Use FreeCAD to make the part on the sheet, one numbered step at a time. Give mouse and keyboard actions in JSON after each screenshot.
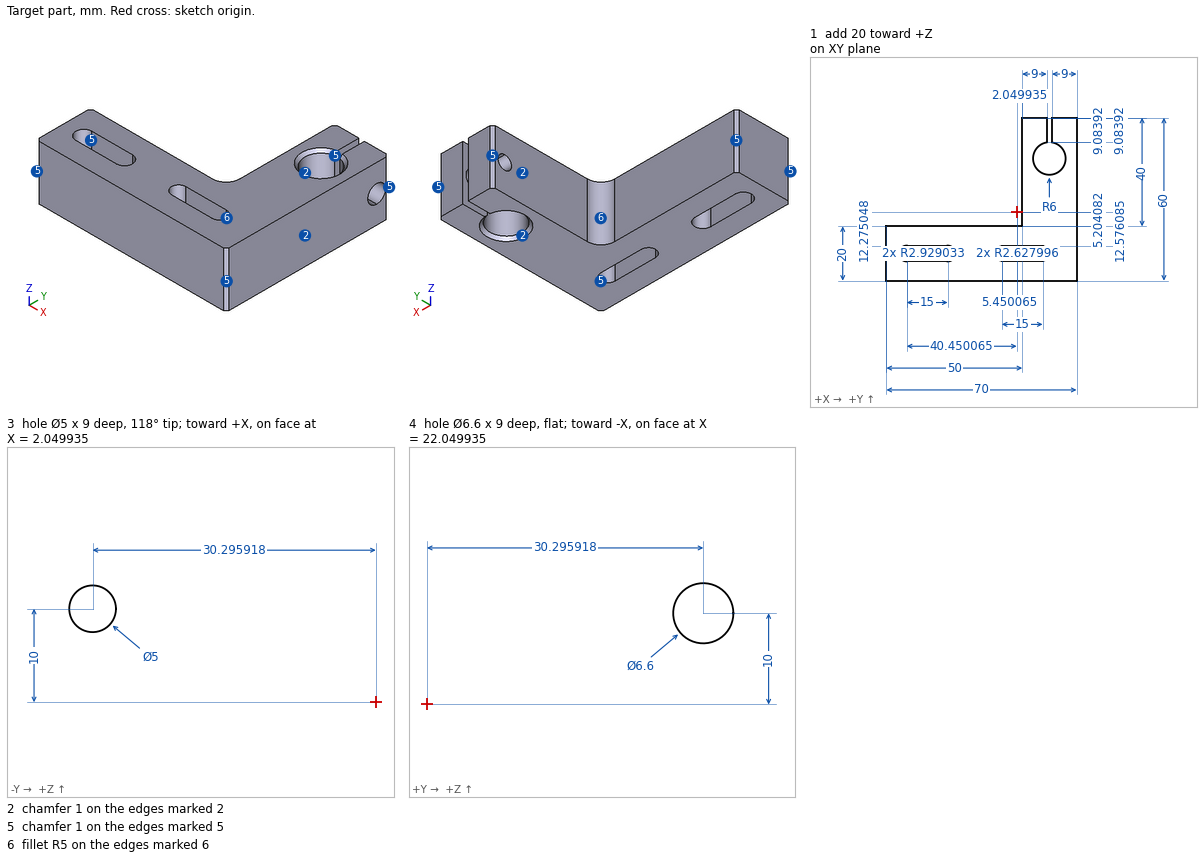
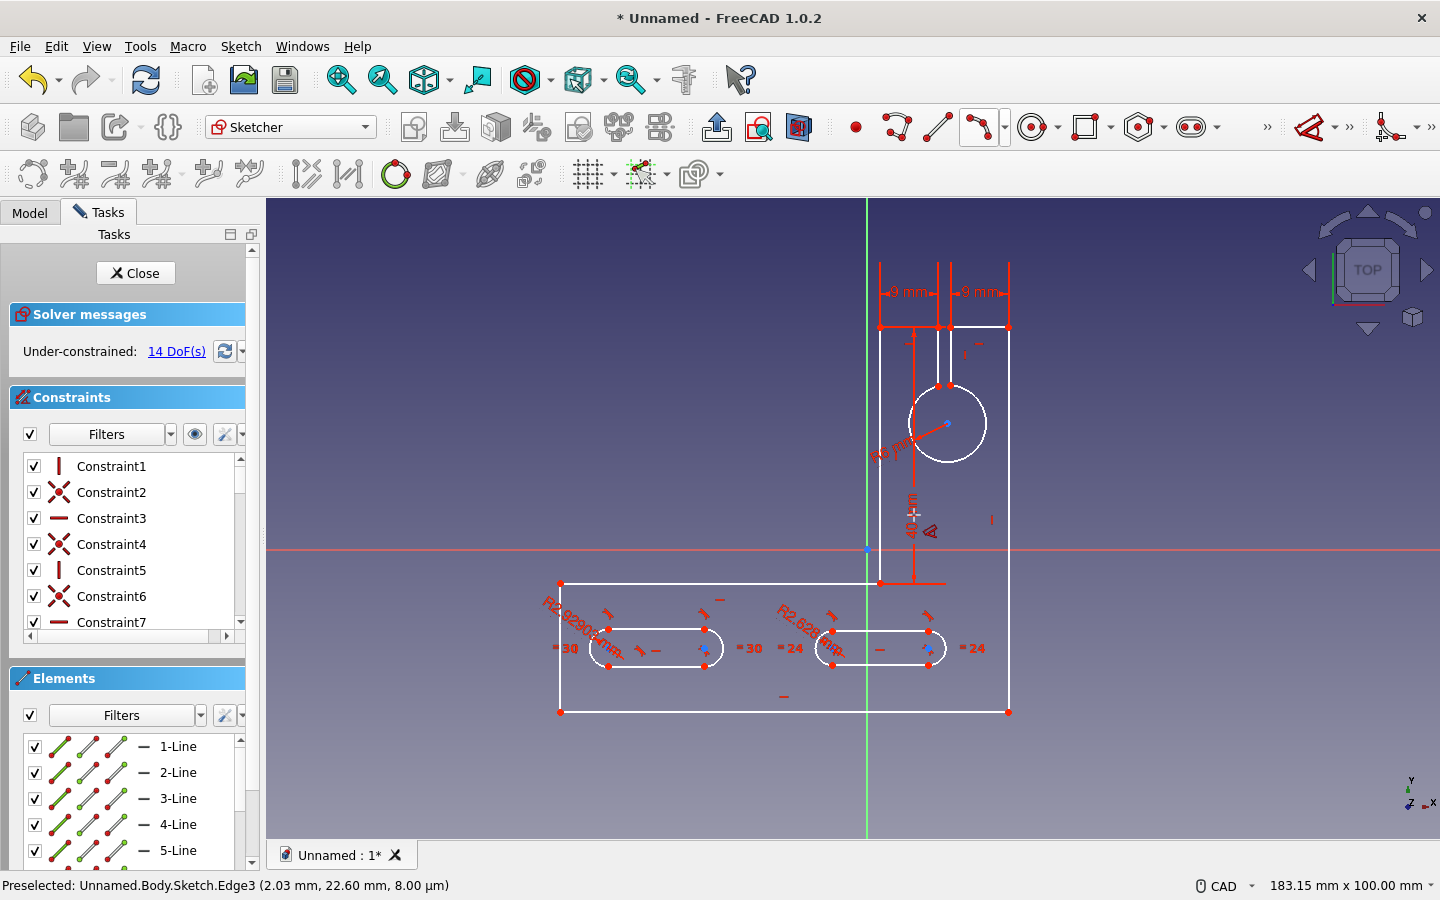
{"action": "left_click", "coordinate": [784, 584]}
{"action": "left_click", "coordinate": [720, 618]}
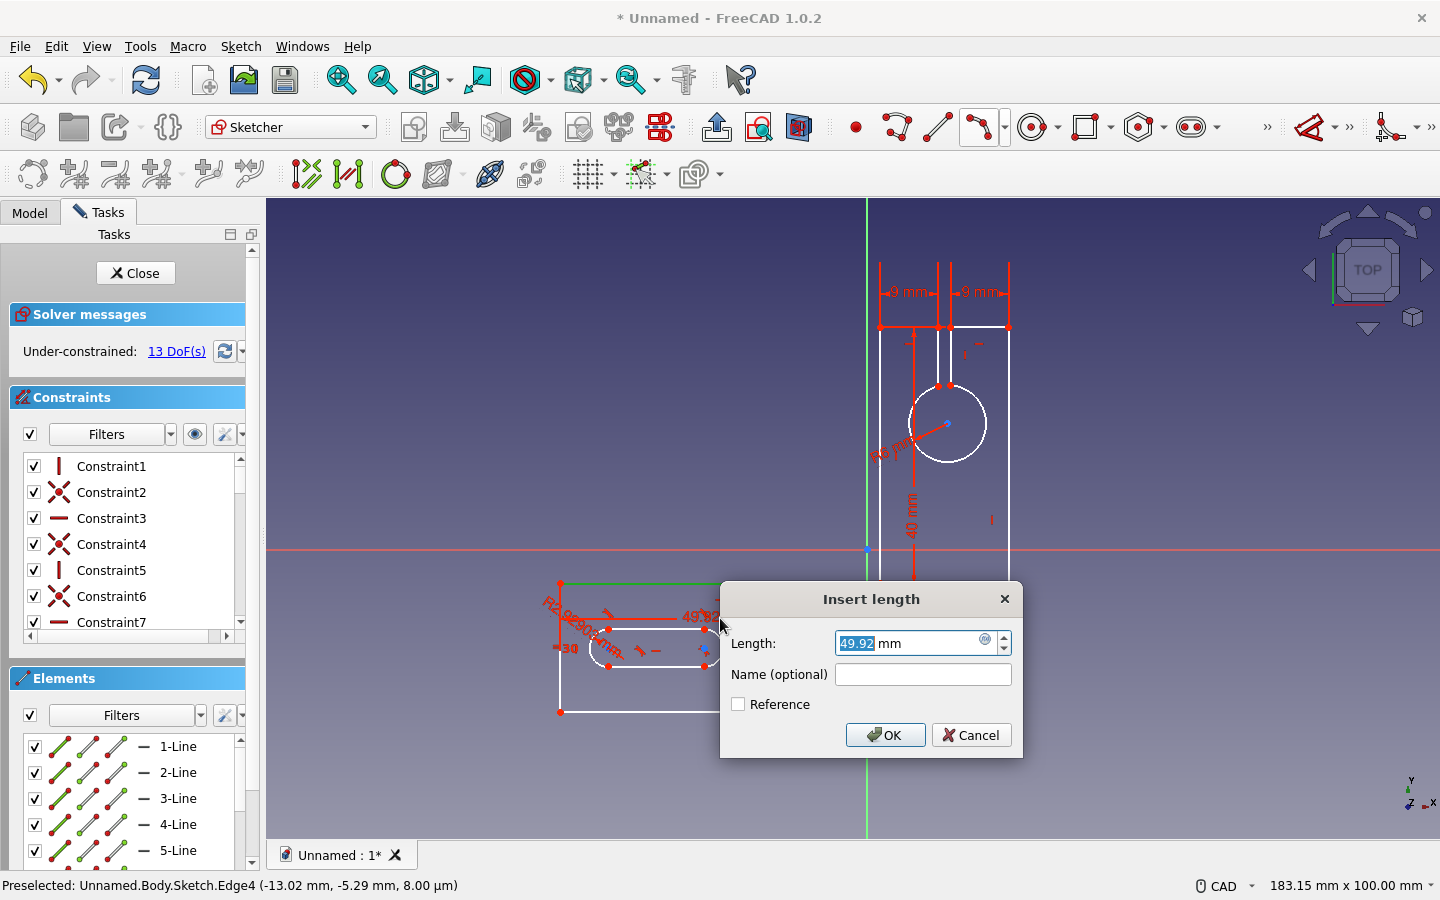
{"action": "type", "text": "50"}
{"action": "key", "text": "Return"}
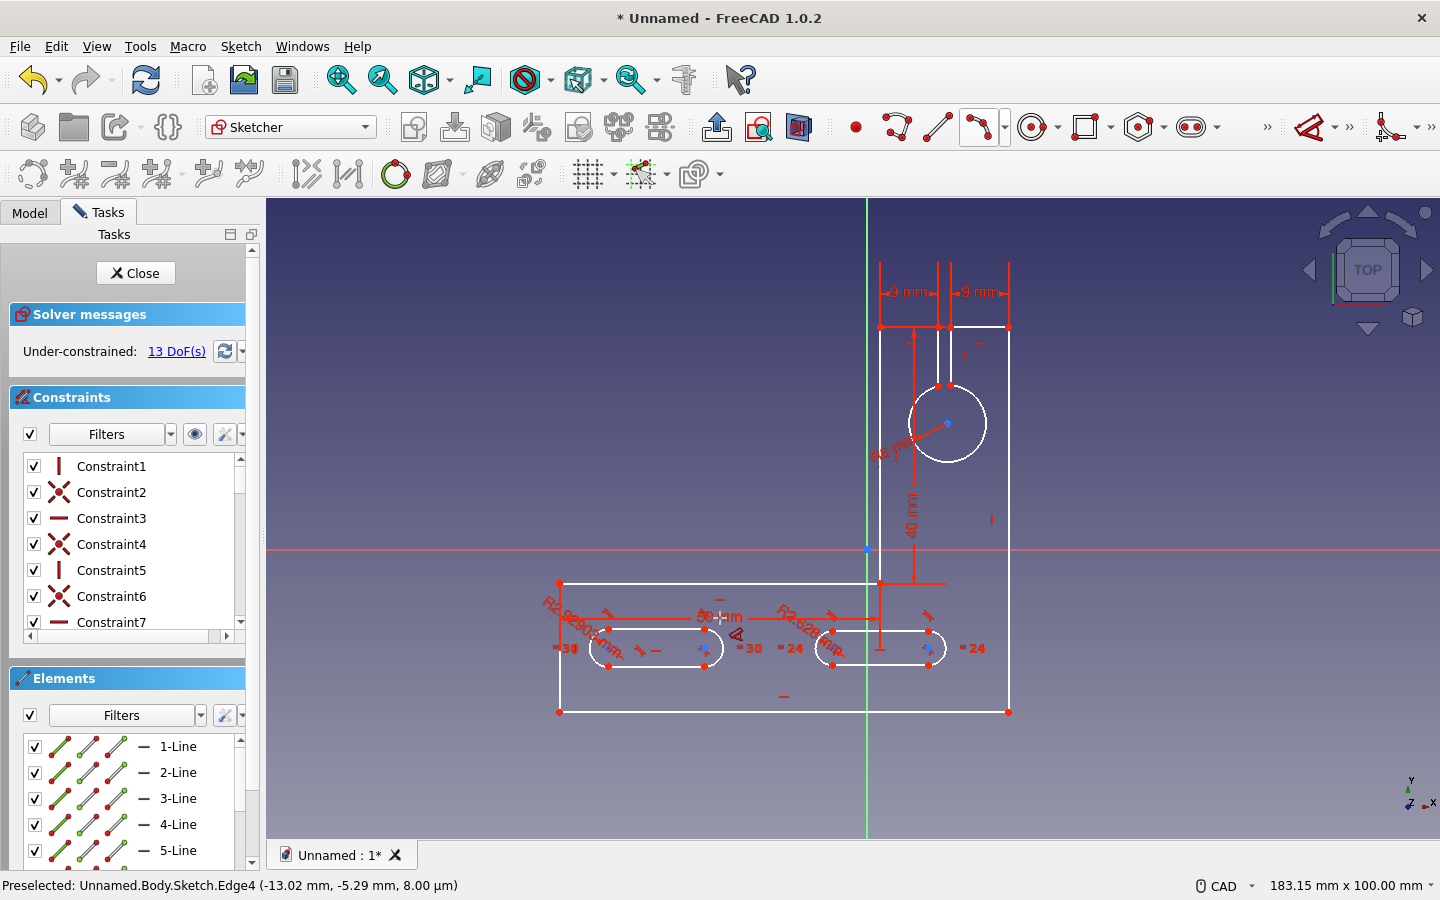
{"action": "left_click", "coordinate": [560, 622]}
{"action": "left_click", "coordinate": [526, 678]}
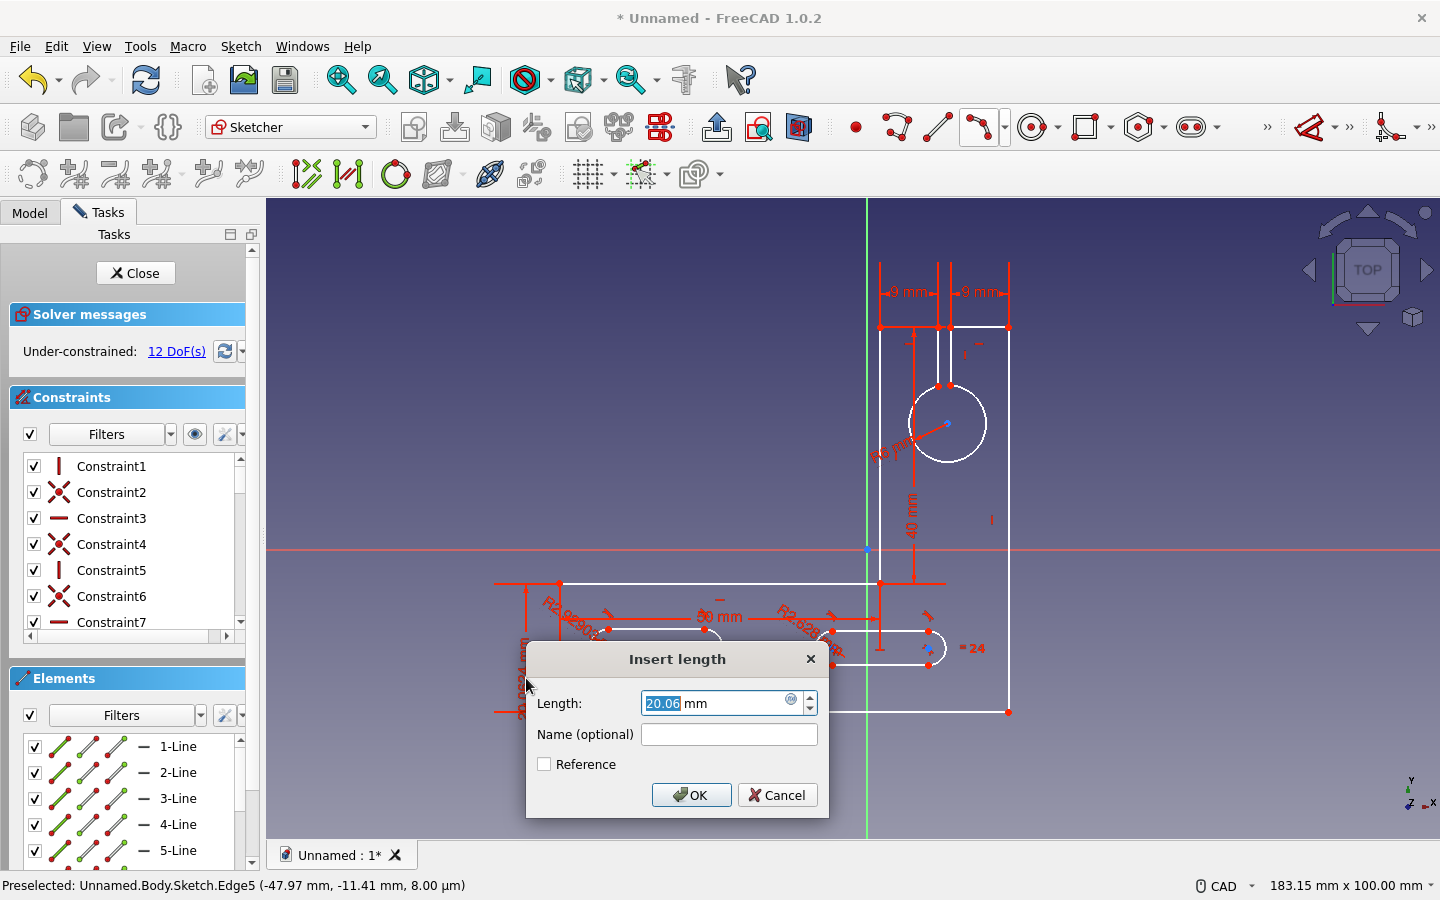
{"action": "type", "text": "20"}
{"action": "key", "text": "Return"}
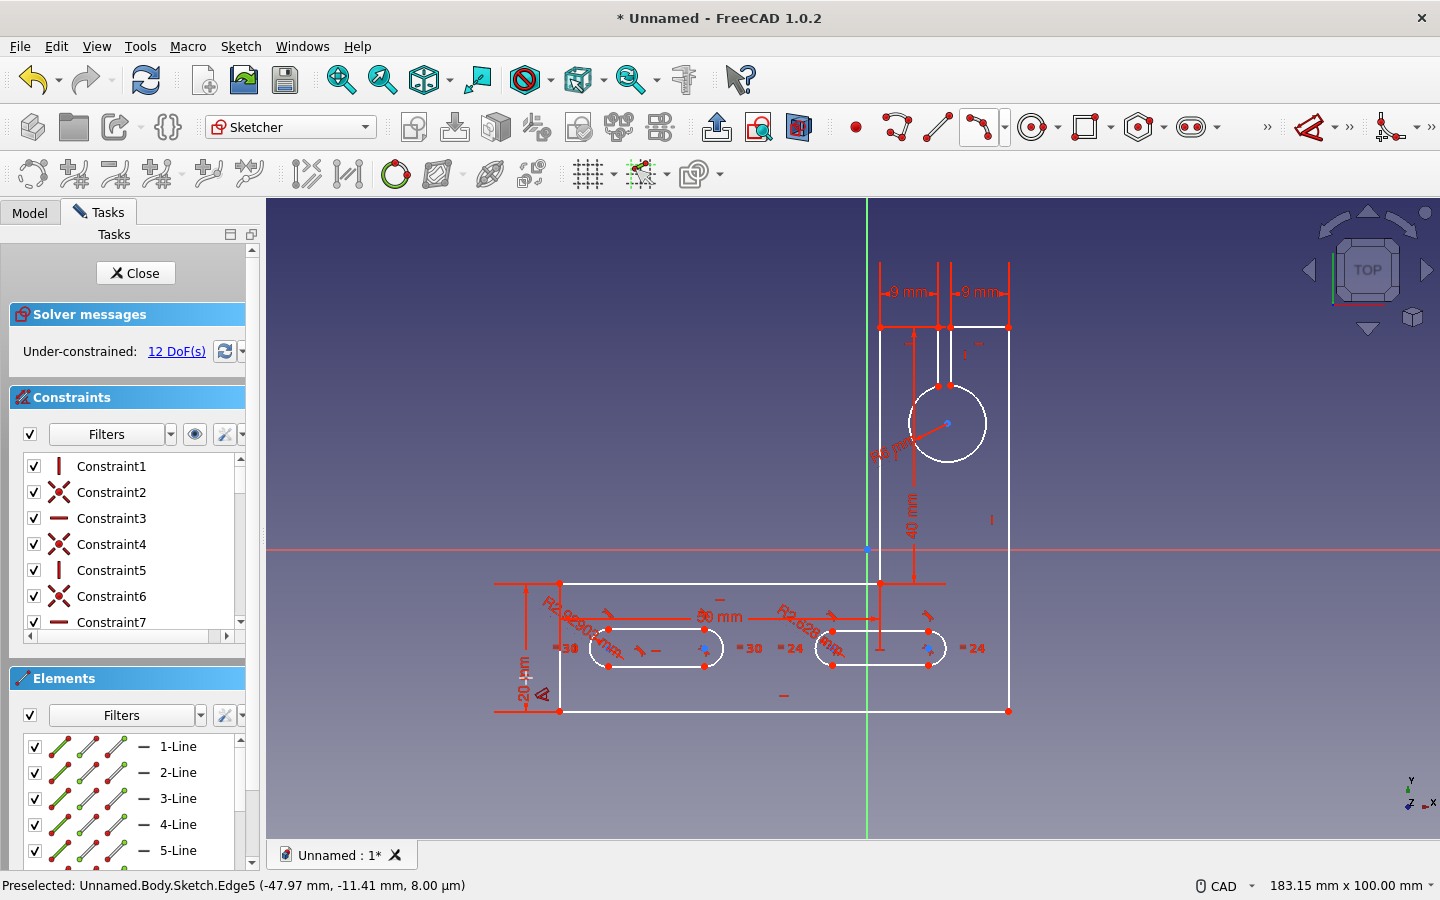
{"action": "left_click", "coordinate": [695, 712]}
{"action": "left_click", "coordinate": [784, 746]}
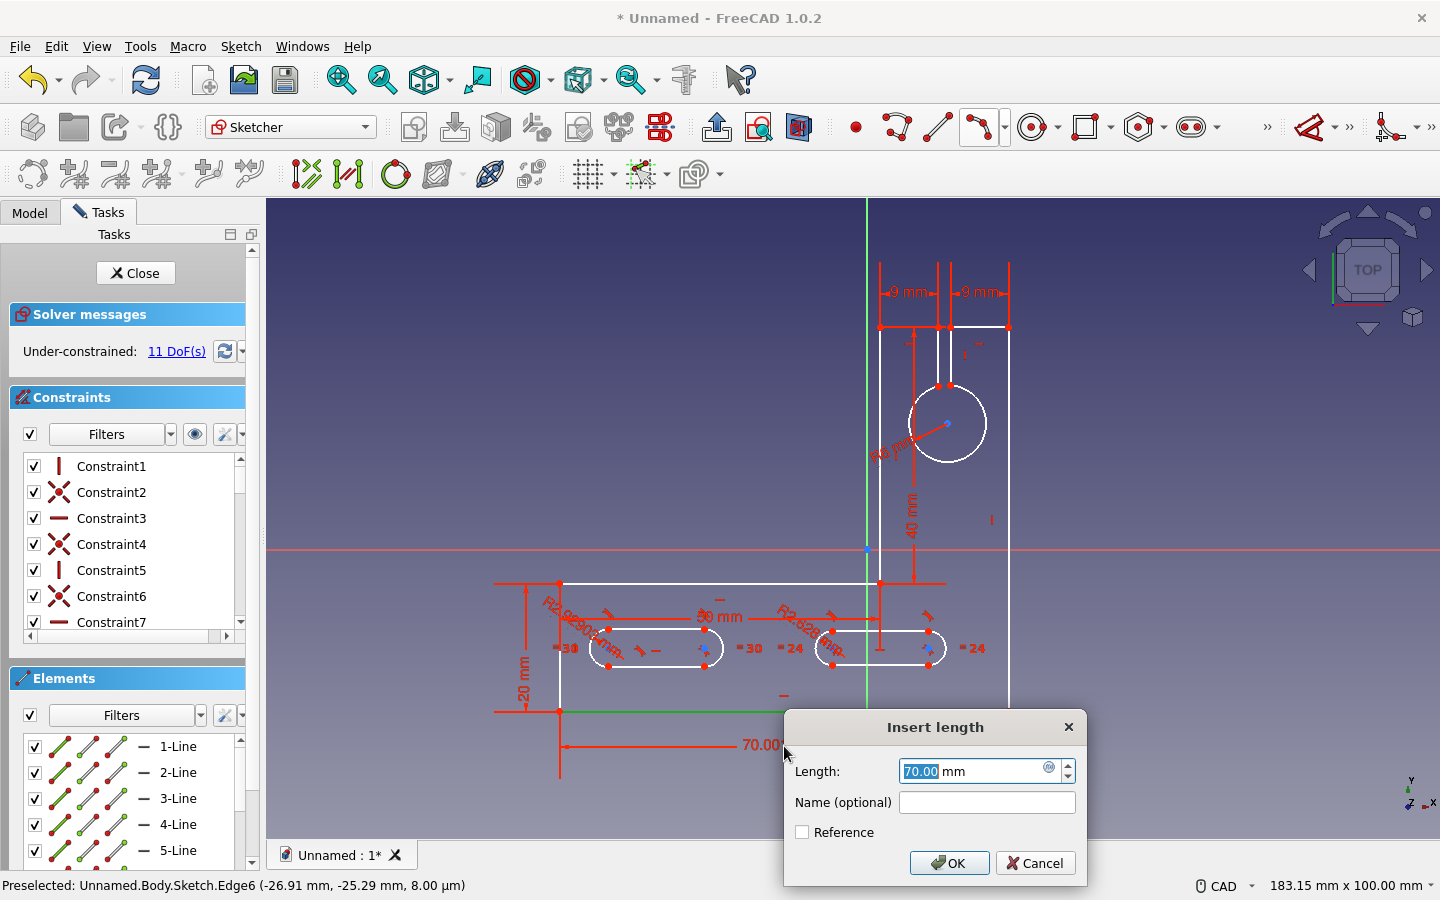
{"action": "type", "text": "70"}
{"action": "key", "text": "Return"}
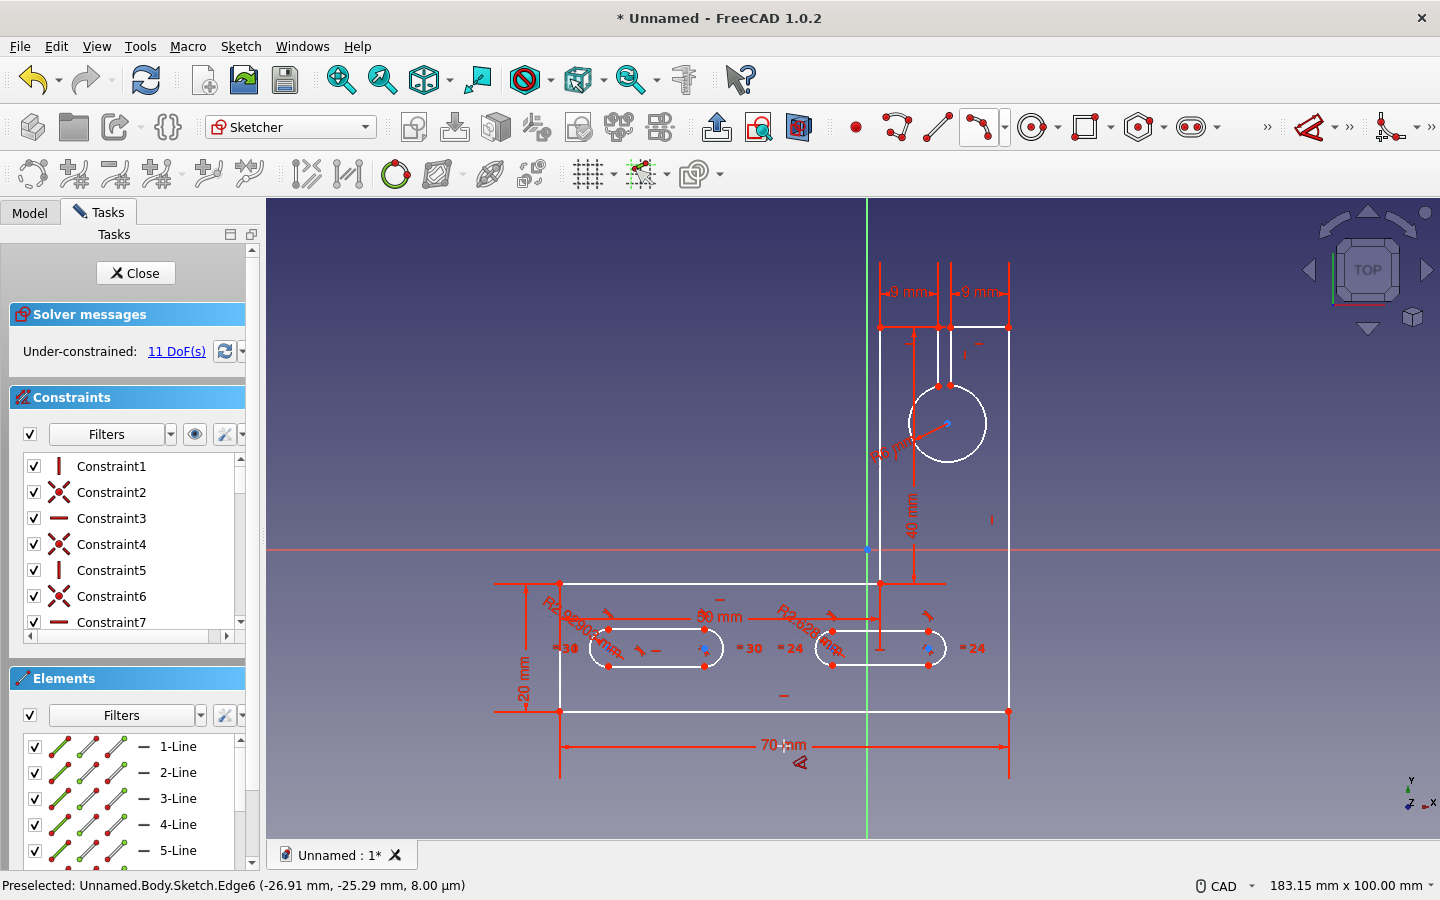
{"action": "left_click", "coordinate": [1009, 597]}
{"action": "left_click", "coordinate": [1043, 520]}